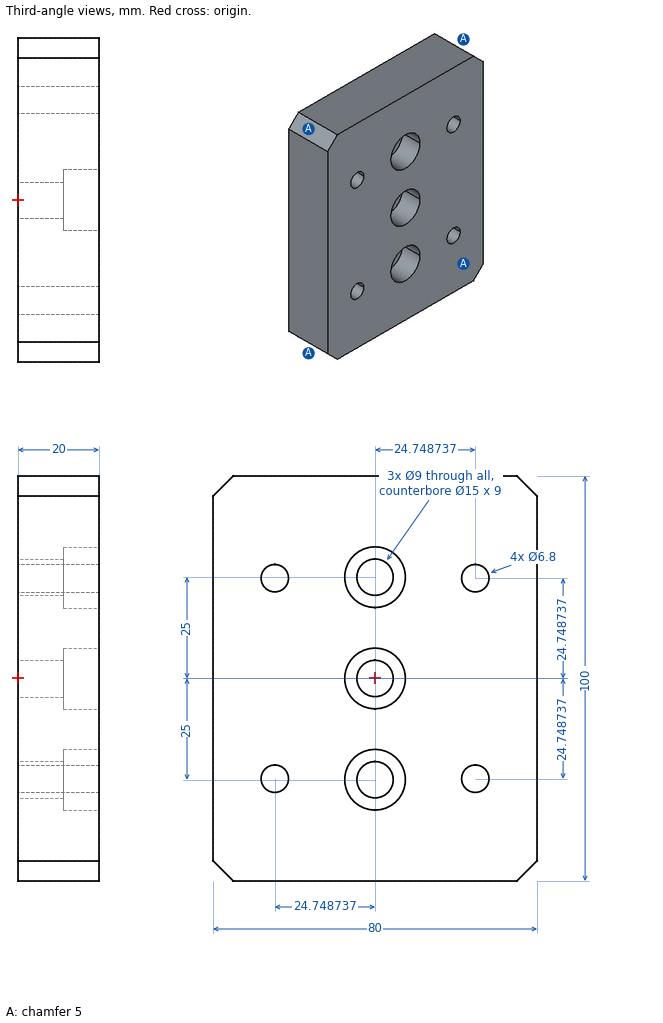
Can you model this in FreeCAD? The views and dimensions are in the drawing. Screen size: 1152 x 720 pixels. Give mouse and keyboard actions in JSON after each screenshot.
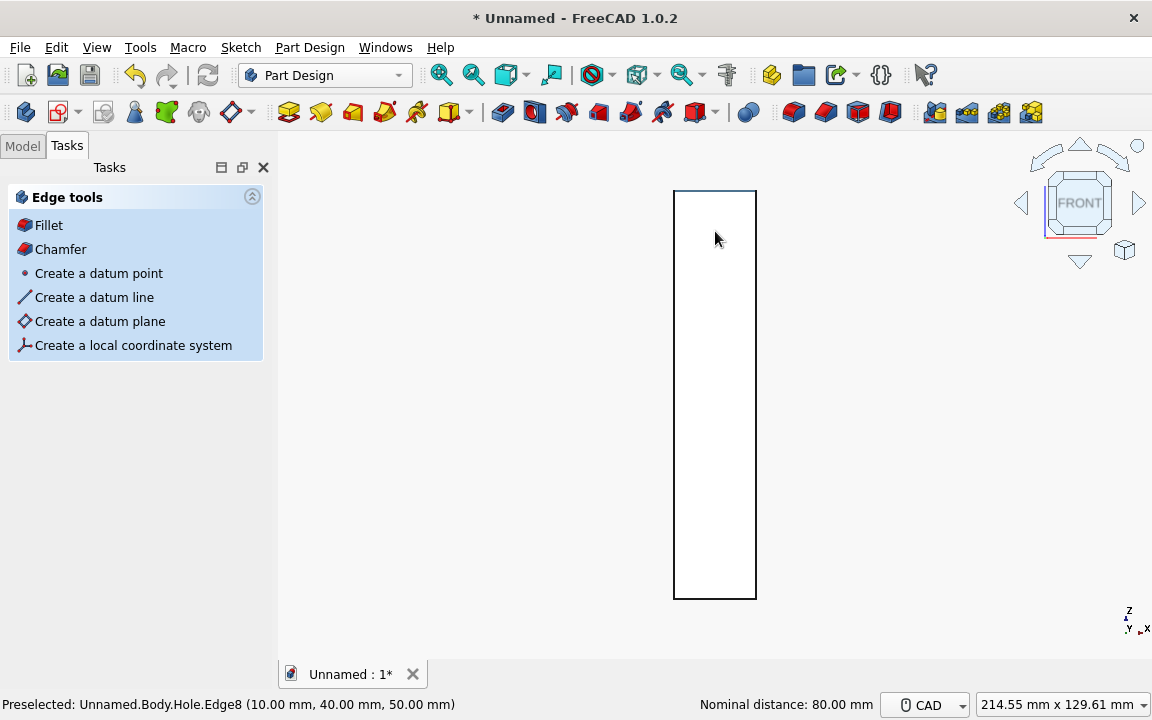
{"action": "left_click", "coordinate": [715, 598], "text": "ctrl"}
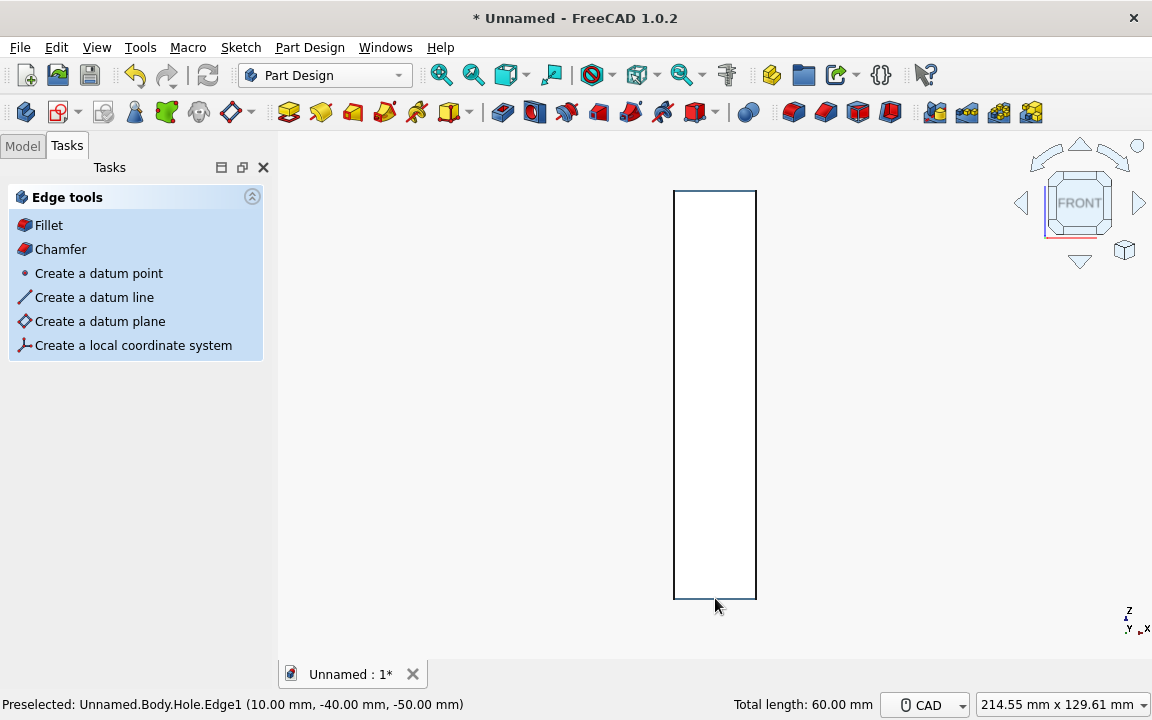
{"action": "key", "text": "3"}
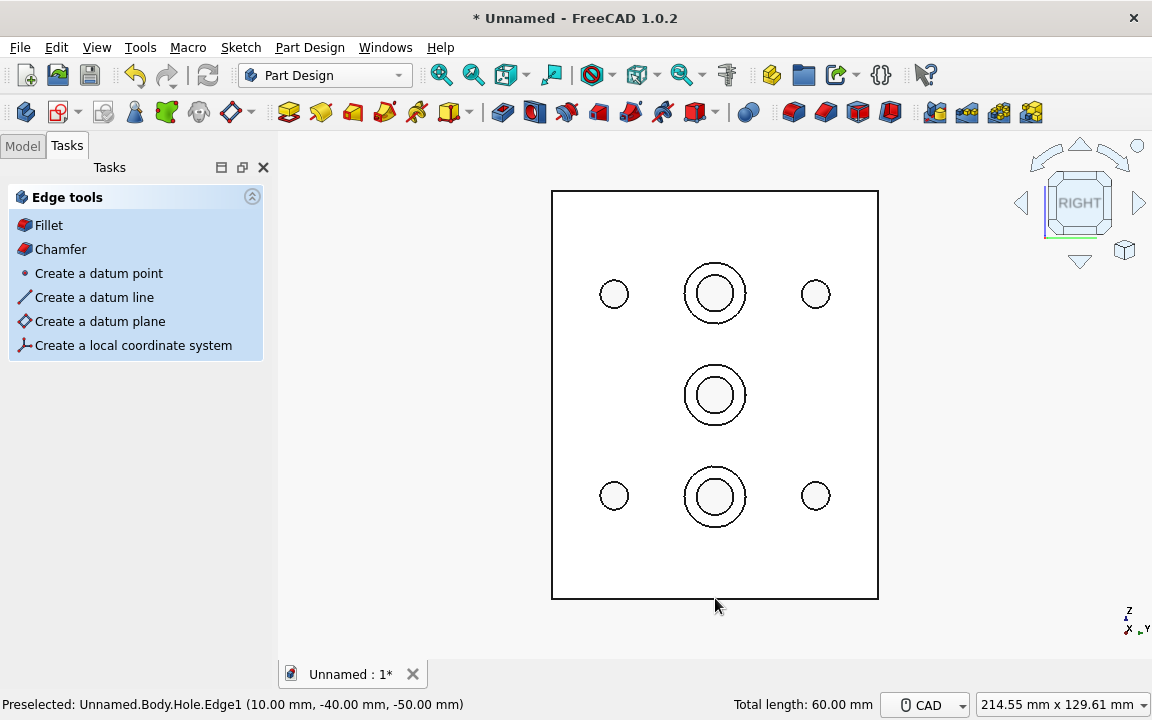
{"action": "key", "text": "5"}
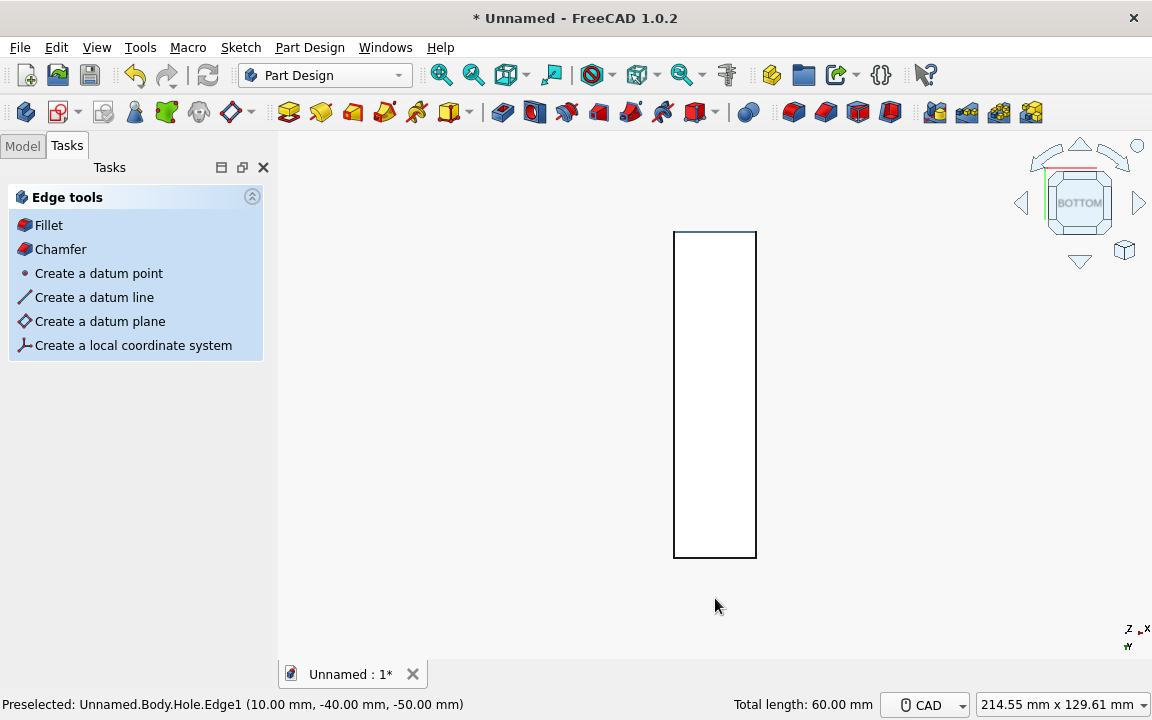
{"action": "left_click", "coordinate": [715, 557], "text": "ctrl"}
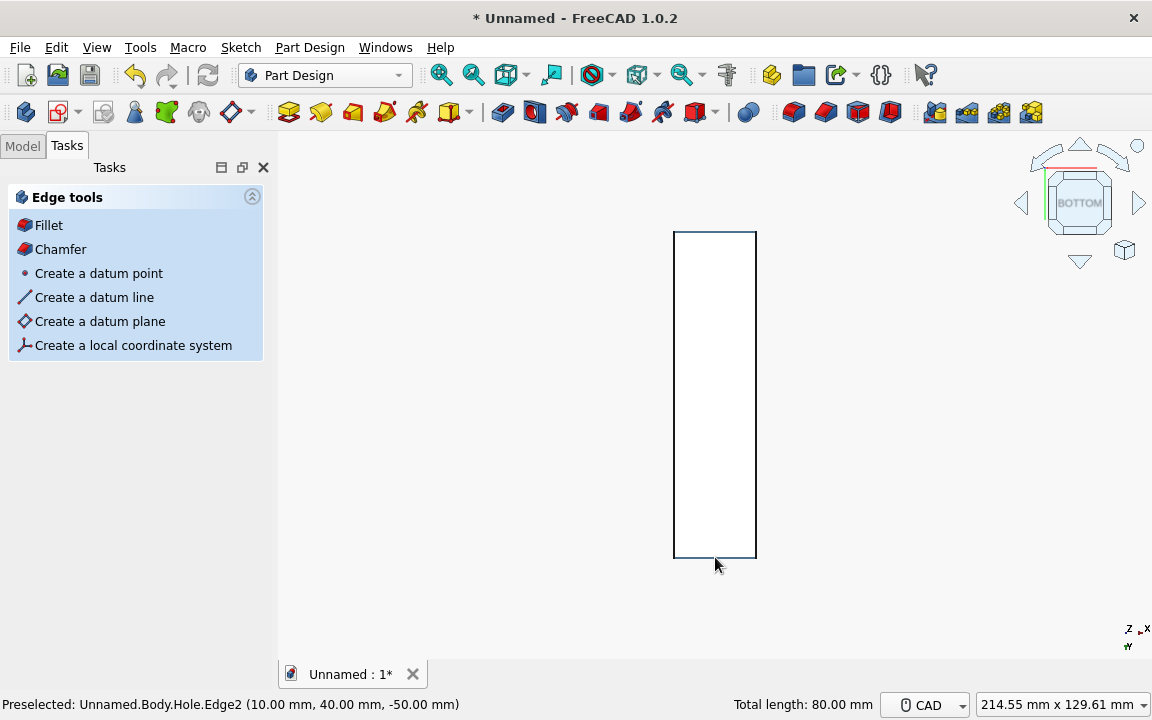
{"action": "left_click", "coordinate": [826, 112]}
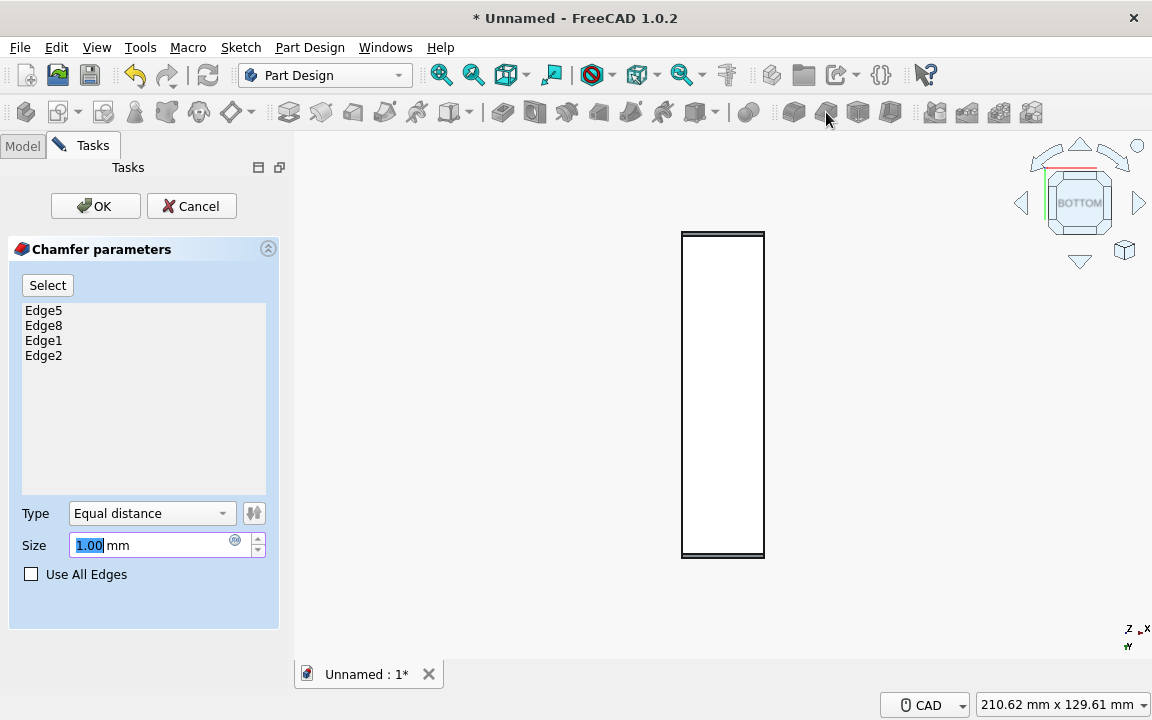
{"action": "type", "text": "5"}
{"action": "key", "text": "Tab"}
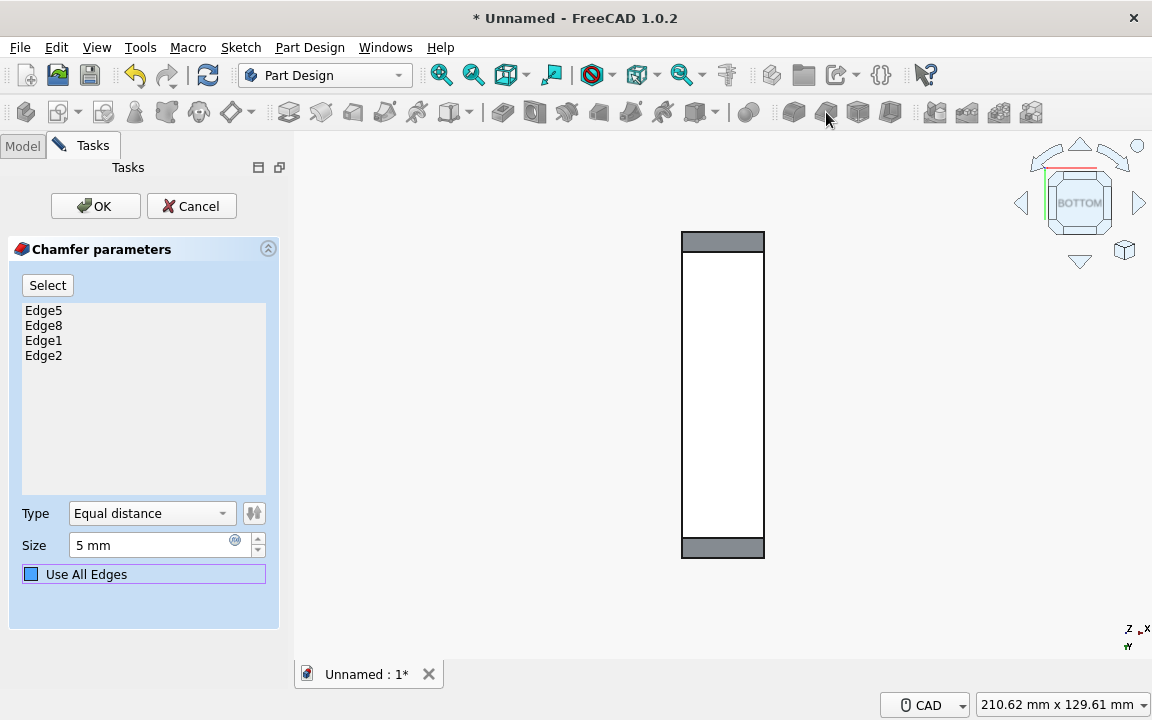
{"action": "left_click", "coordinate": [96, 206]}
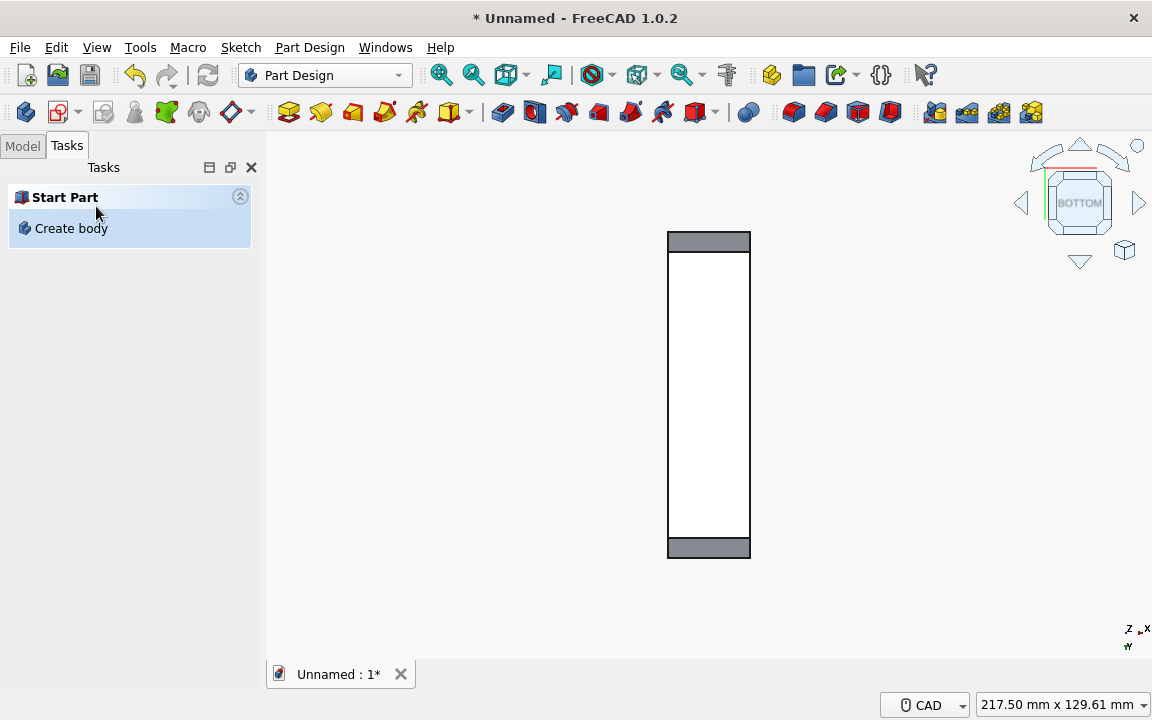
{"action": "key", "text": "0"}